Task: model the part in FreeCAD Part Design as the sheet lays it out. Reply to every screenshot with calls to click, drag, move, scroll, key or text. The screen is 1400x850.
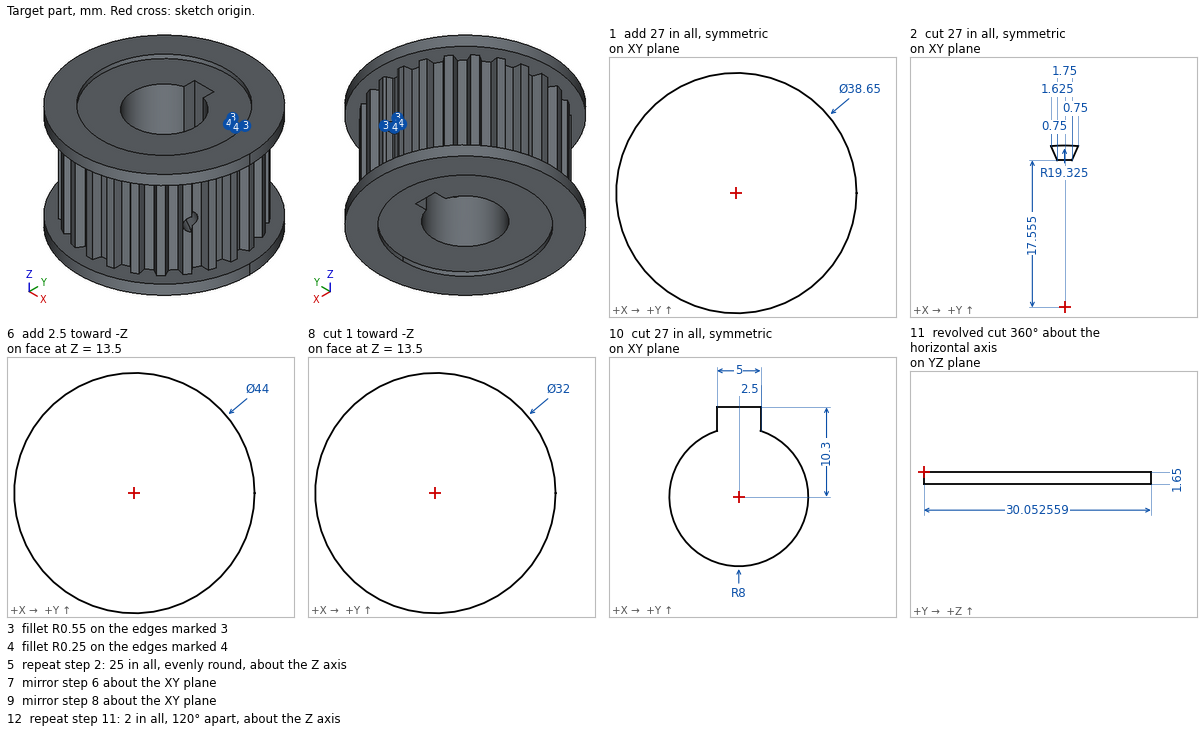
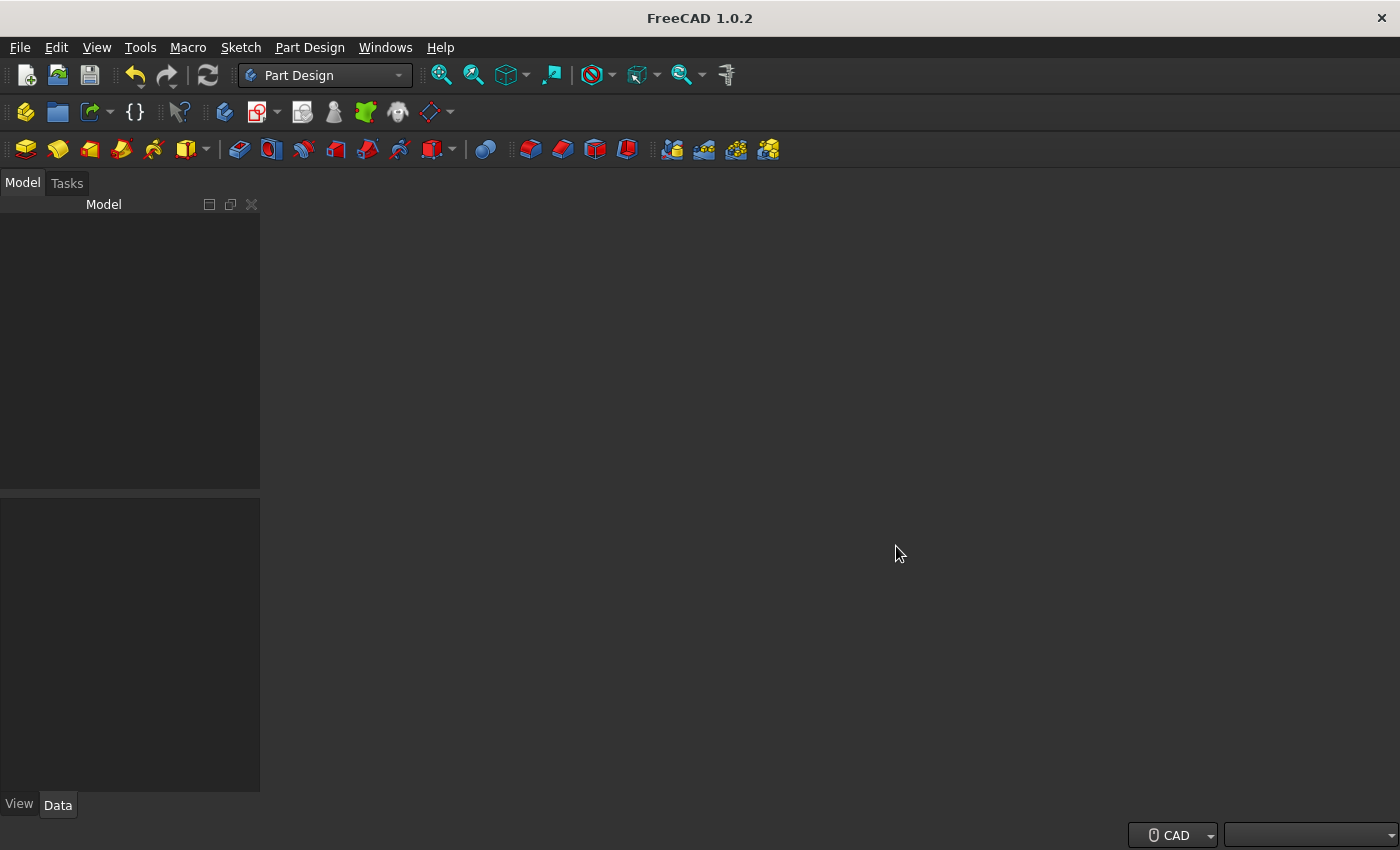
click(26, 76)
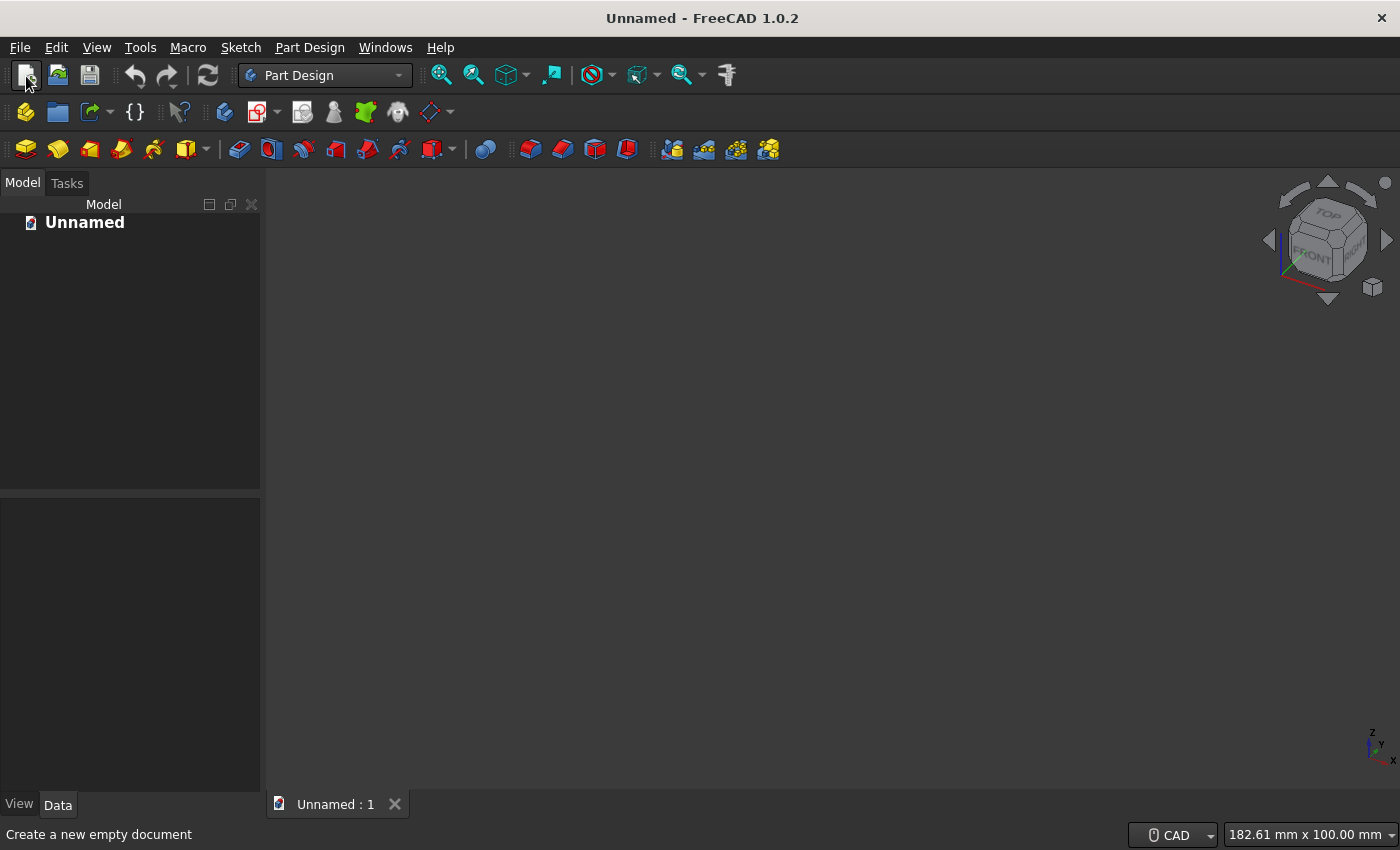
click(258, 112)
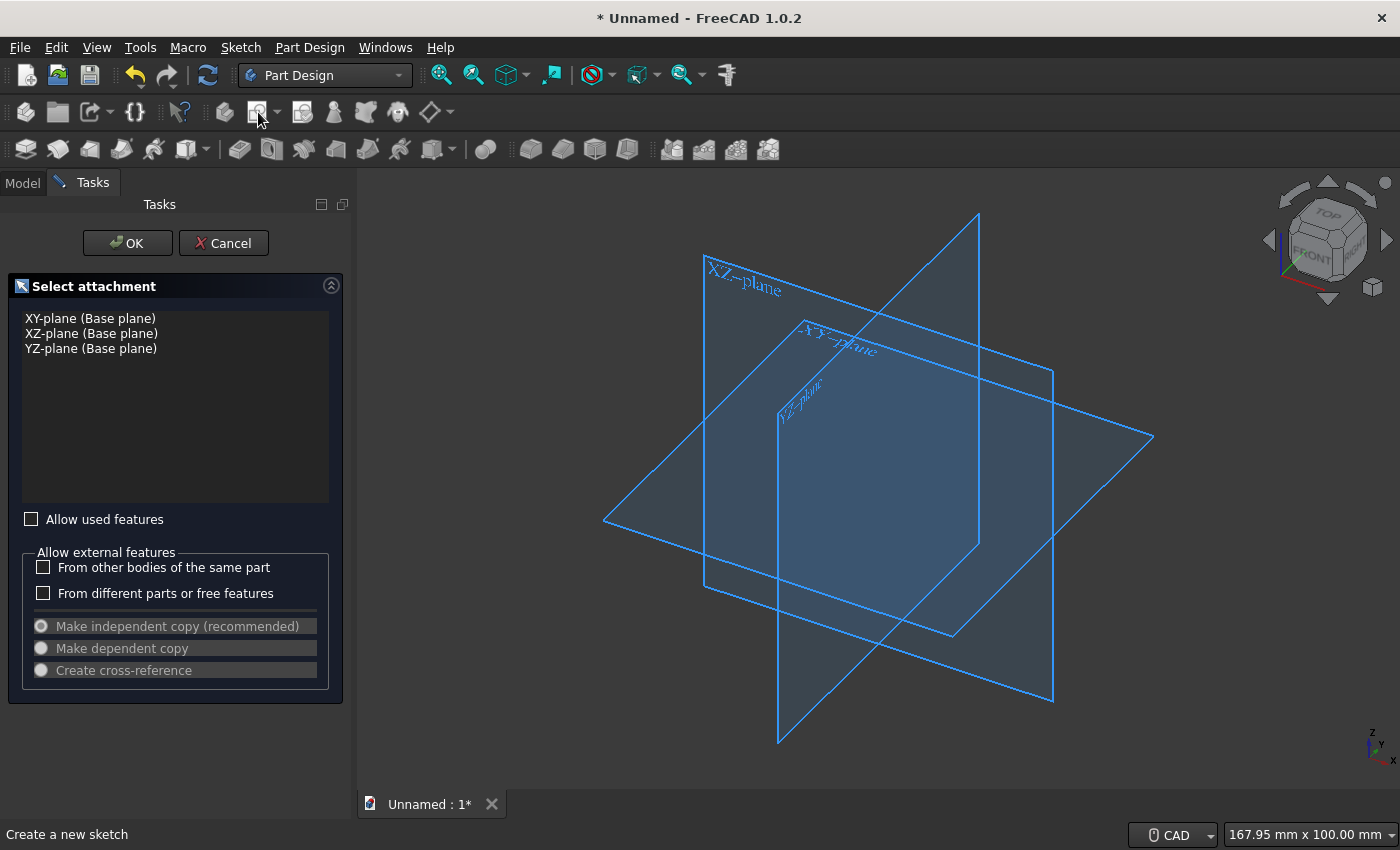
click(82, 318)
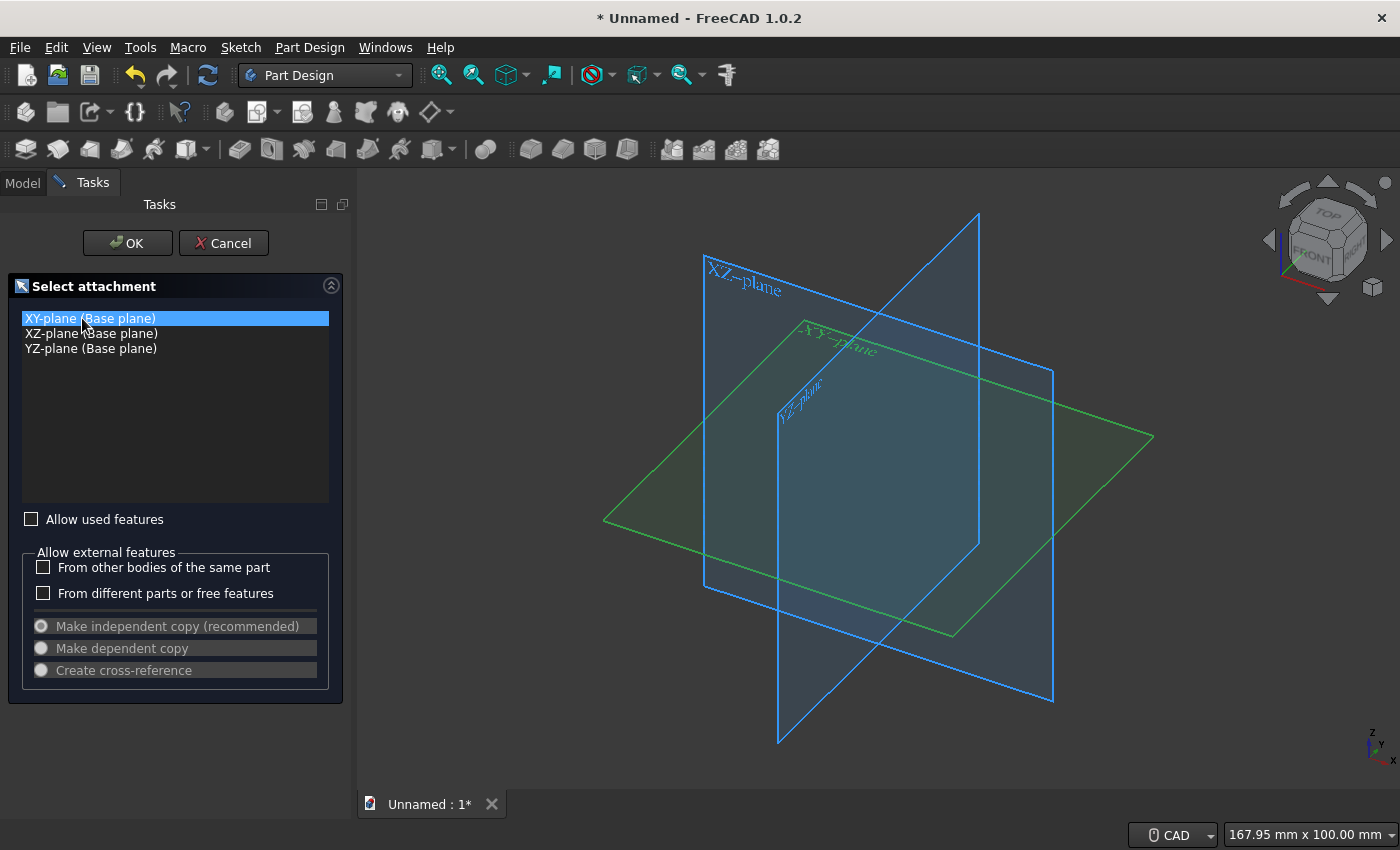
click(128, 243)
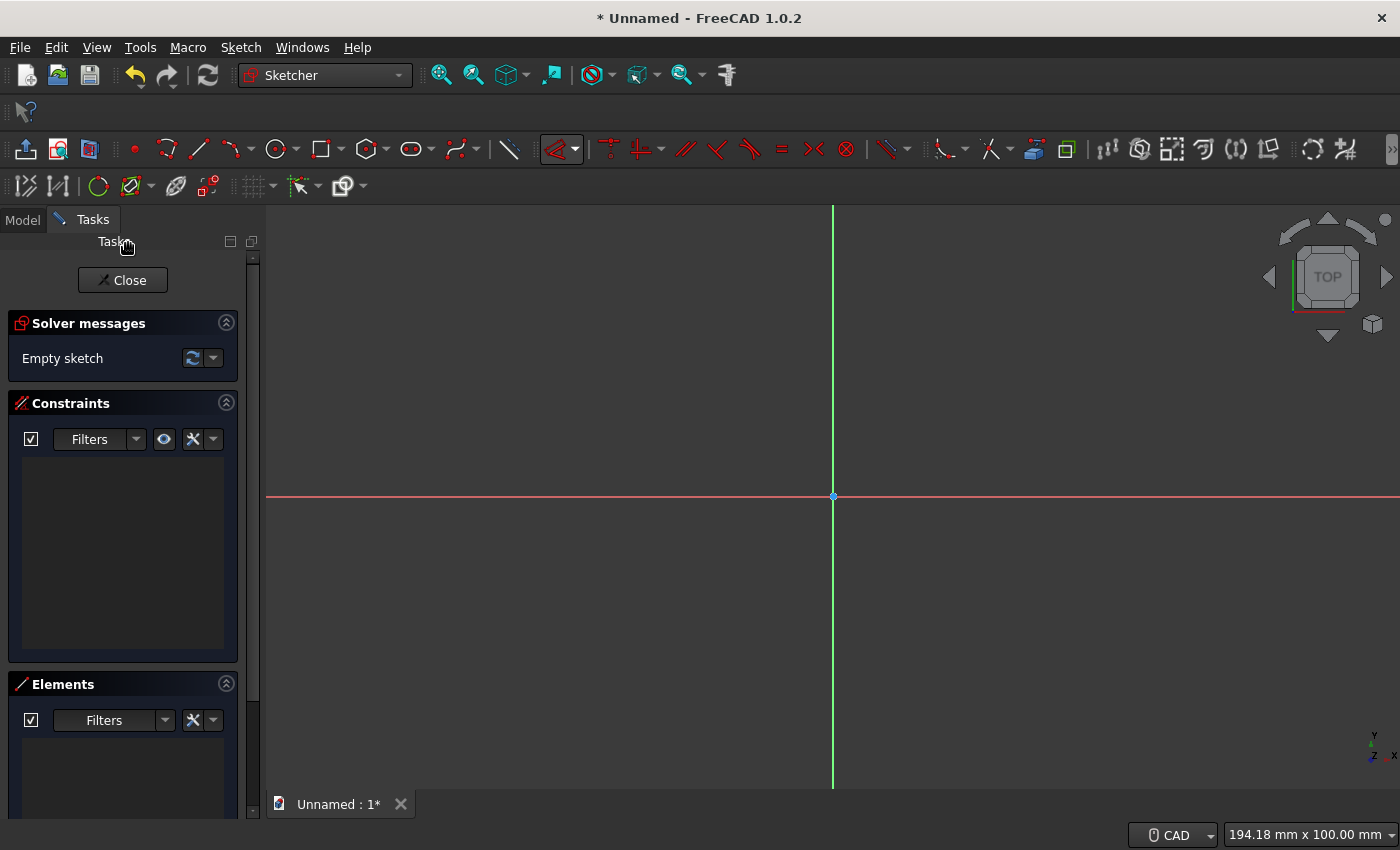
scroll(916, 497, up, 3)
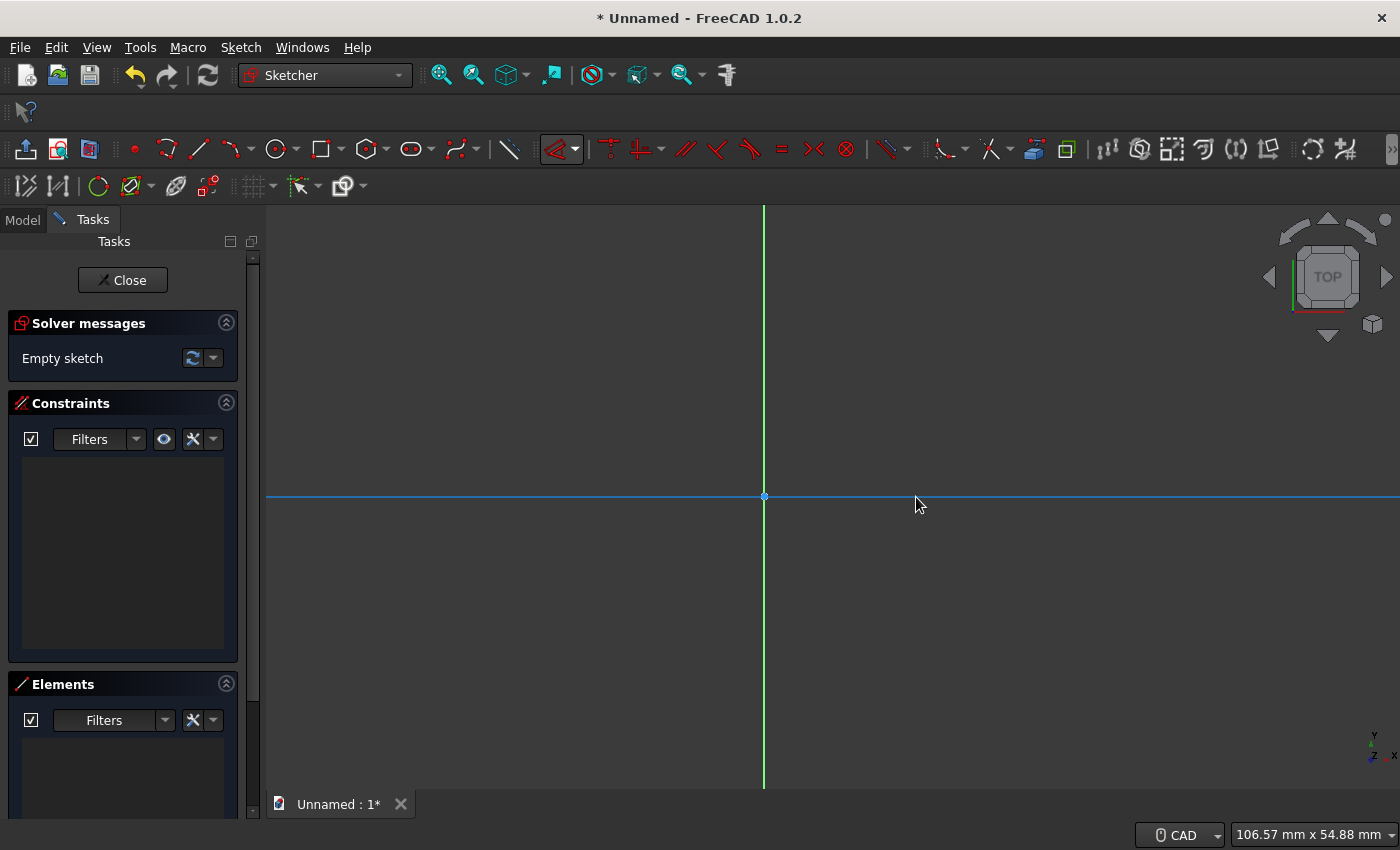
click(276, 150)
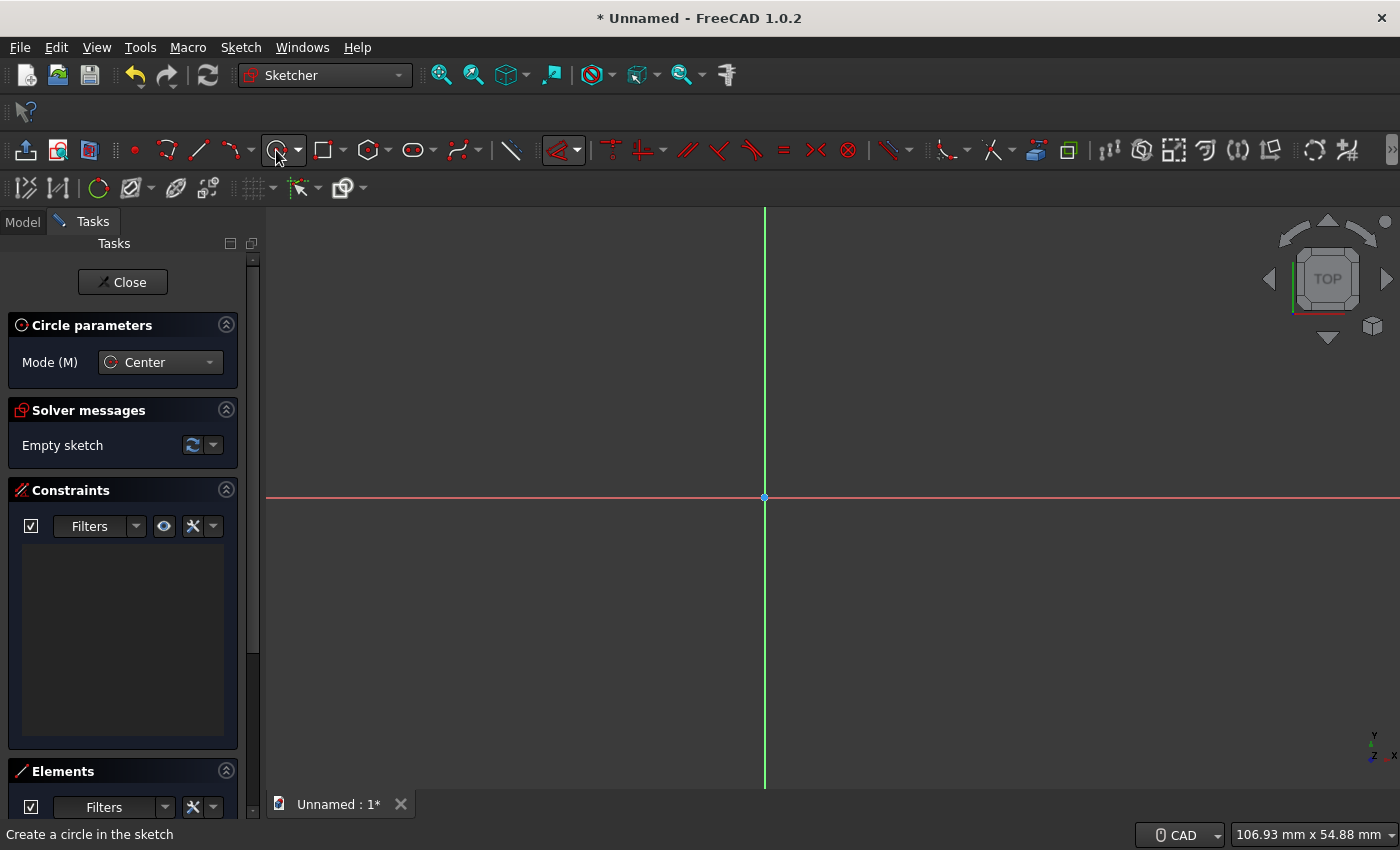
click(765, 498)
move(909, 353)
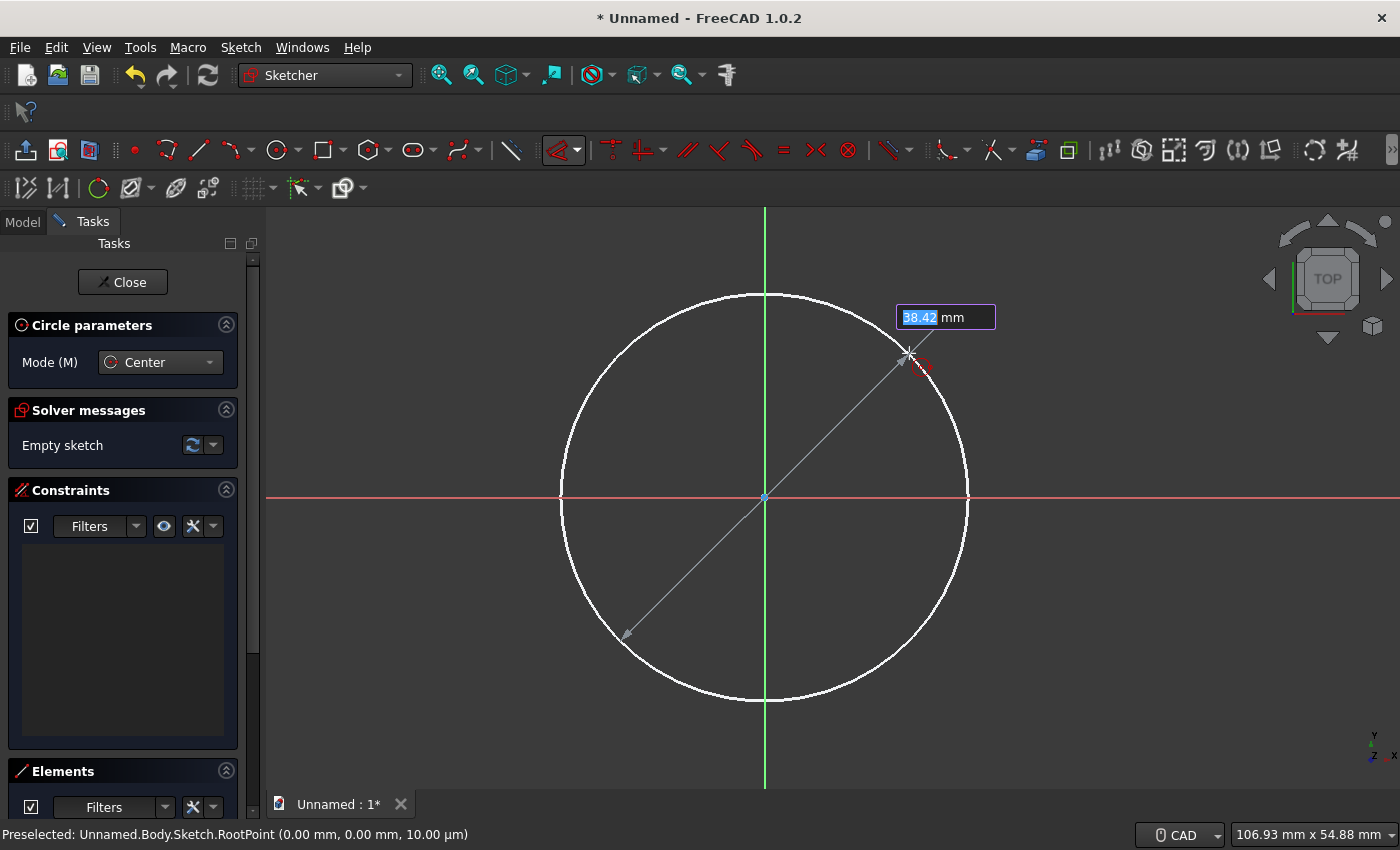
text(38.65)
key(Return)
key(Escape)